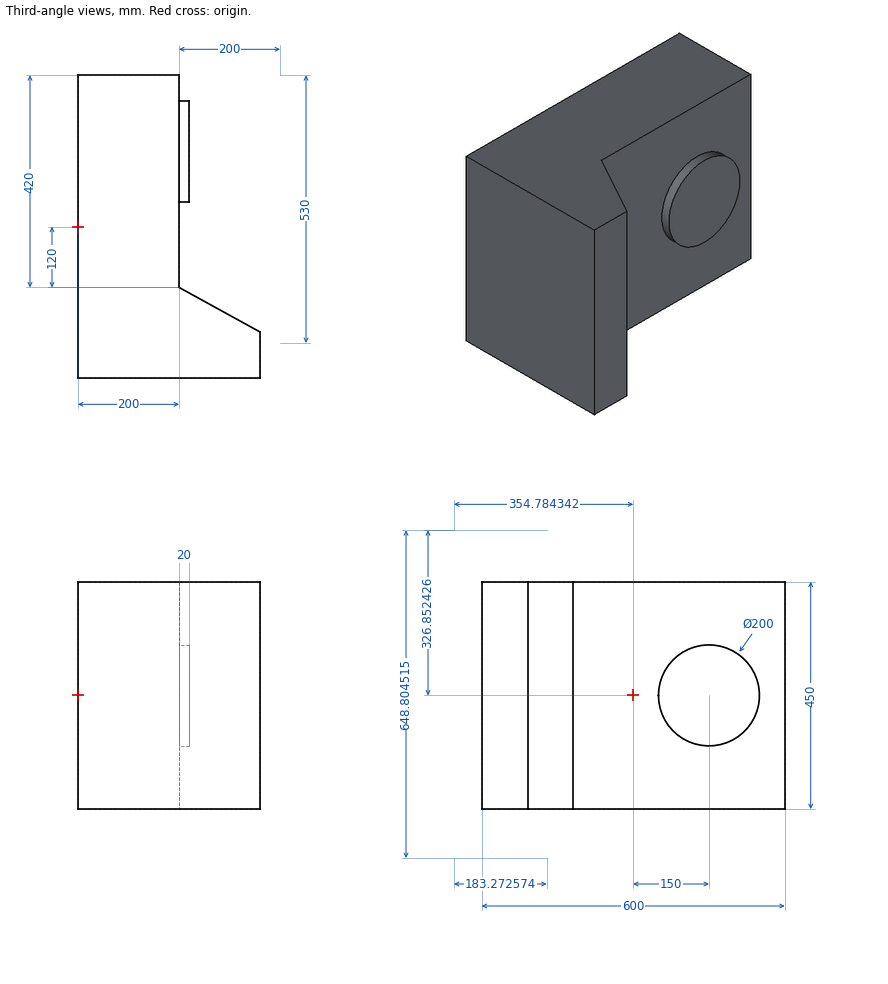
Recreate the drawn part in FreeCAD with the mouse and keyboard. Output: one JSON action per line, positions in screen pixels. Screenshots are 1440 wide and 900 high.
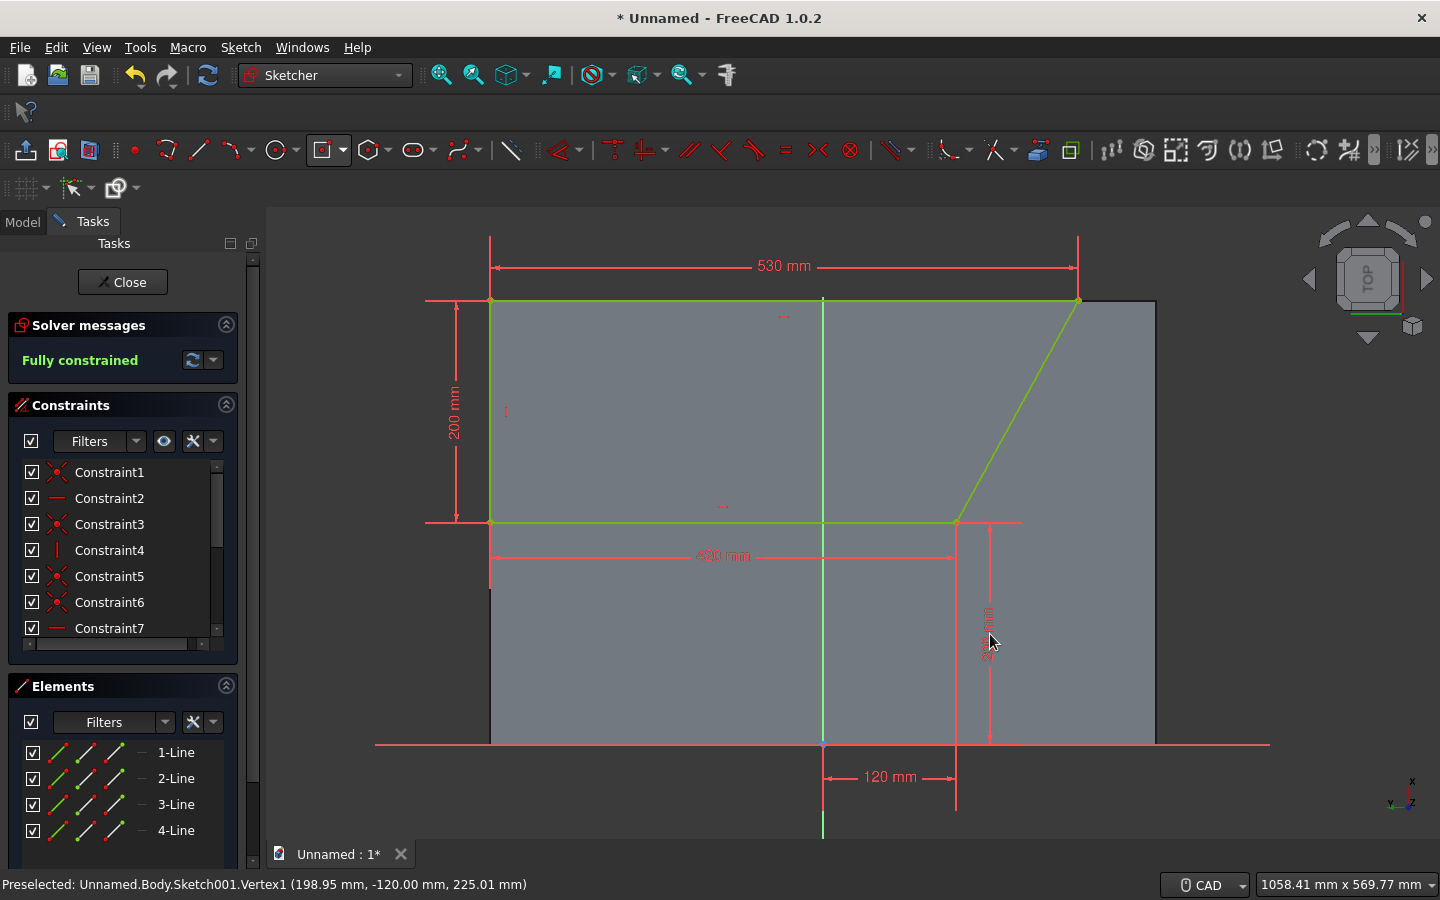
{"action": "left_click", "coordinate": [123, 282]}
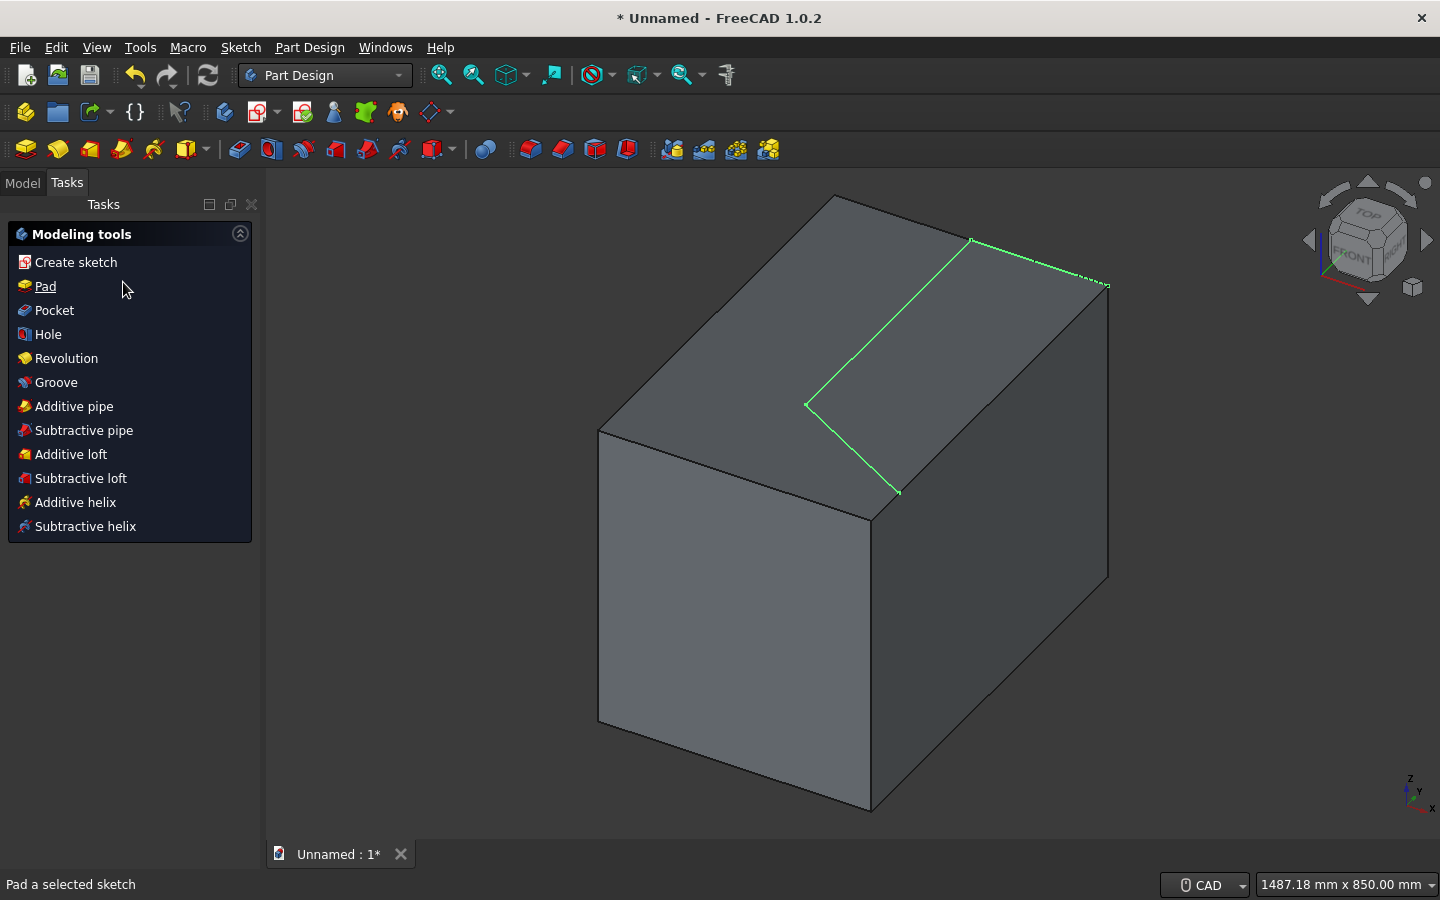
{"action": "left_click", "coordinate": [240, 150]}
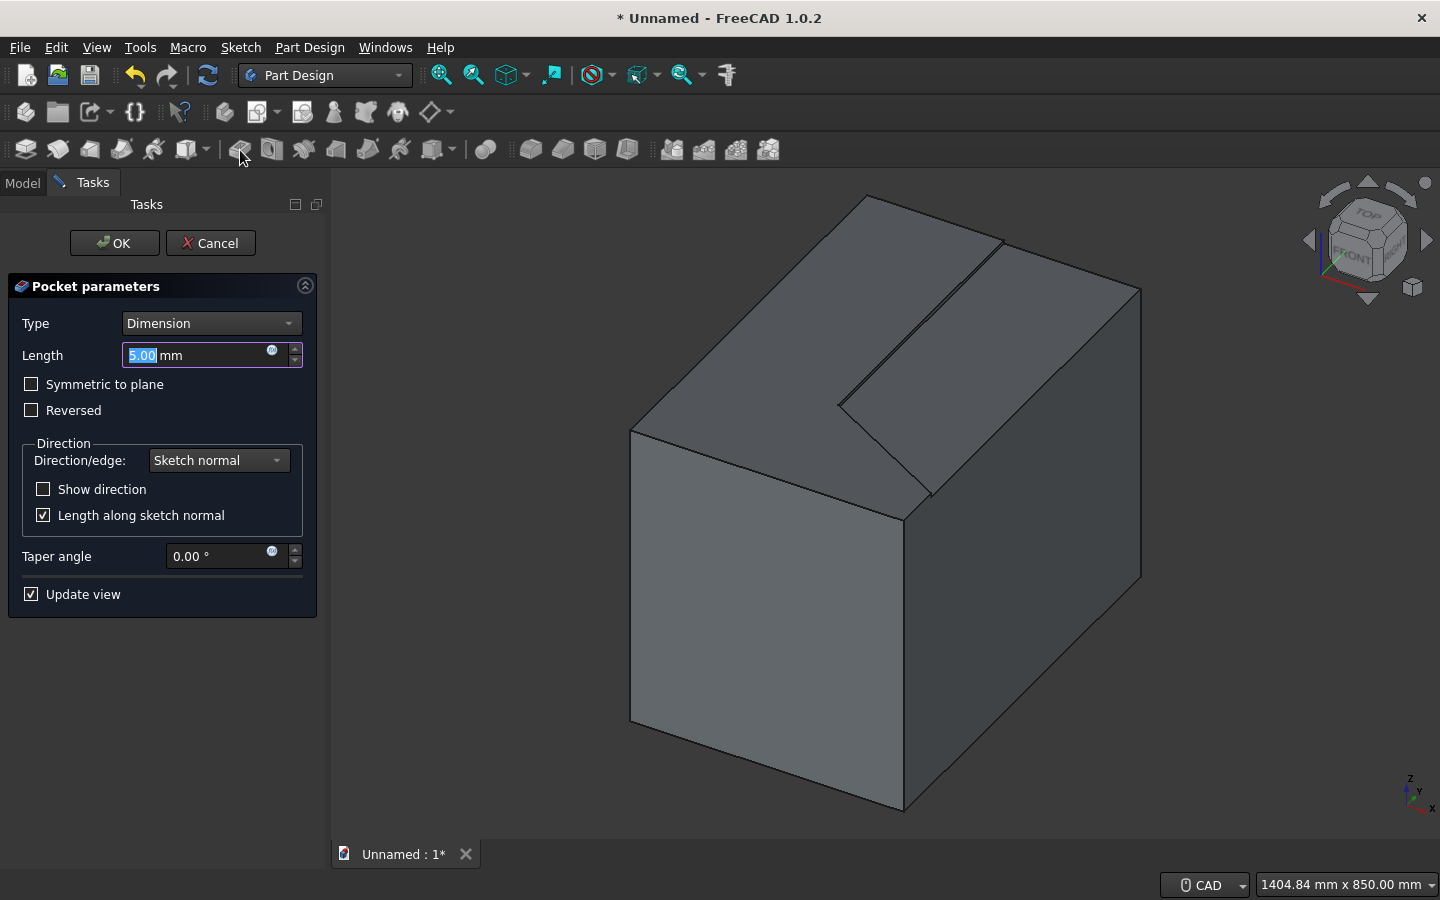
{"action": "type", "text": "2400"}
{"action": "key", "text": "Tab"}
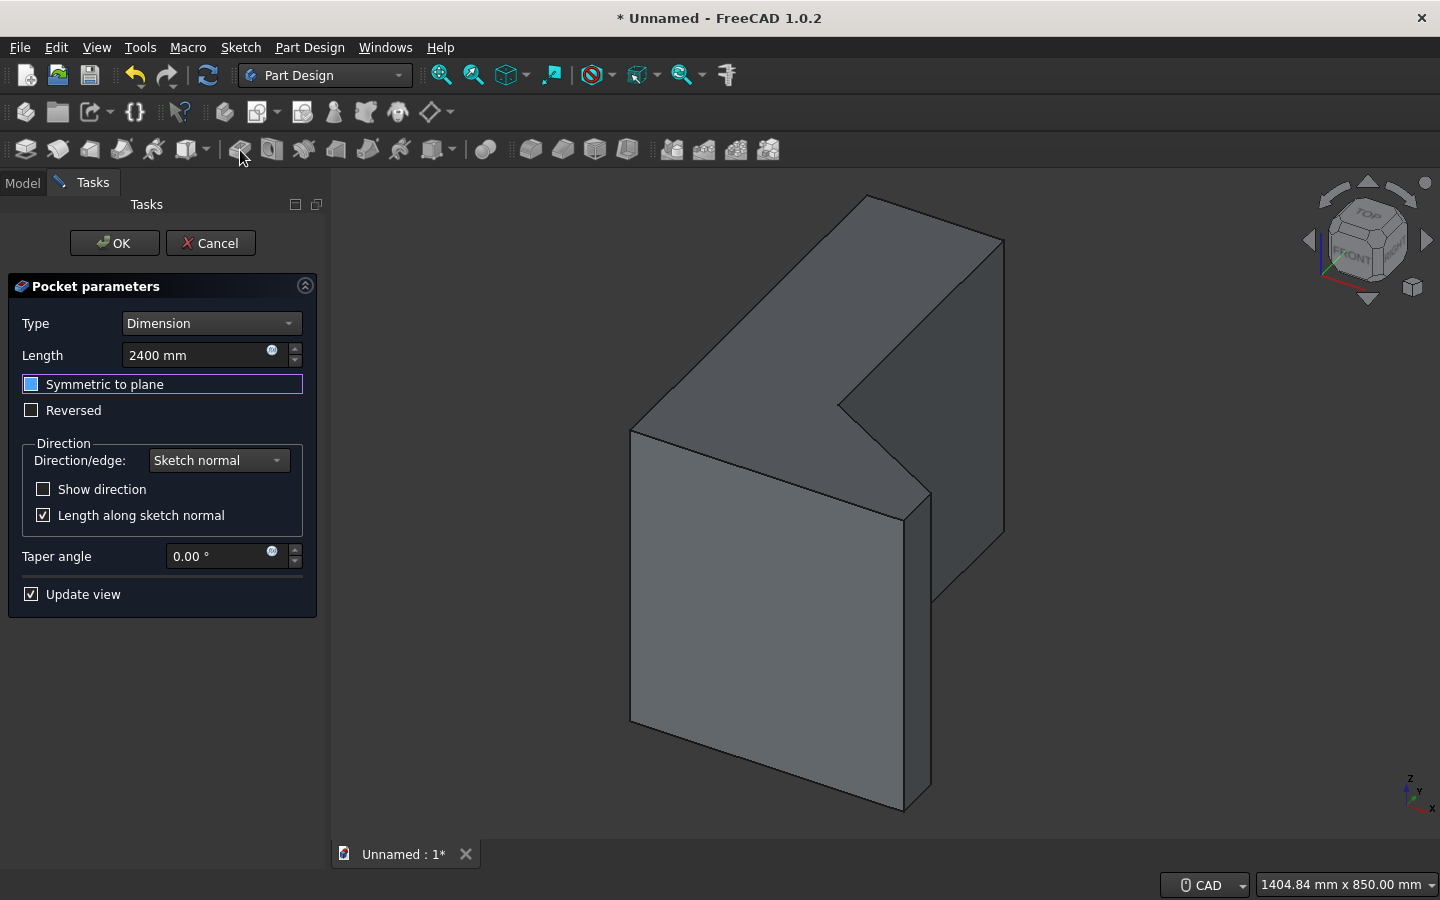
{"action": "left_click", "coordinate": [115, 243]}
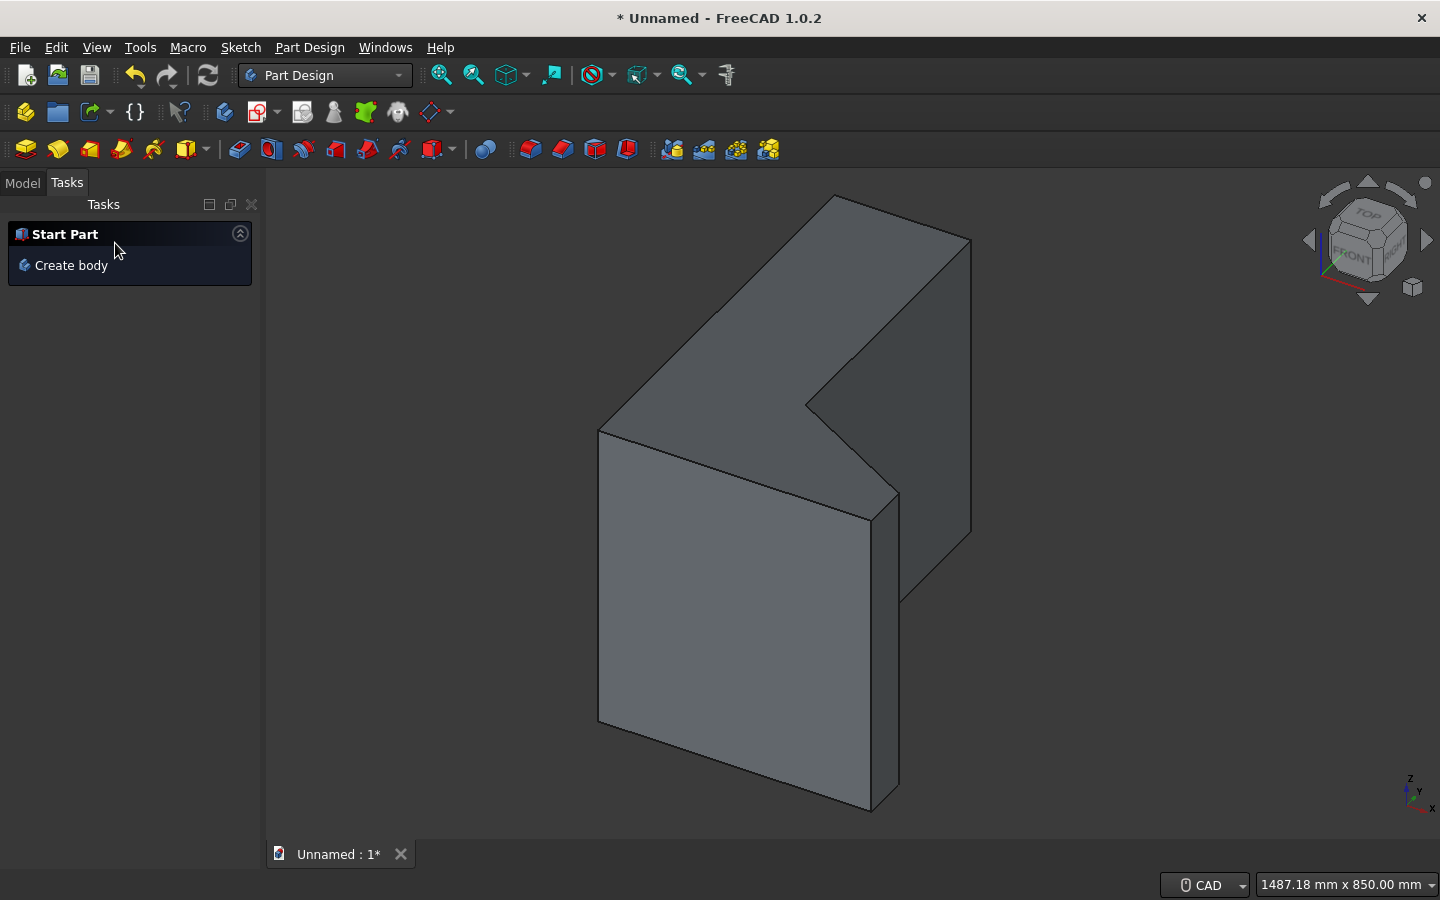
{"action": "left_click", "coordinate": [885, 693]}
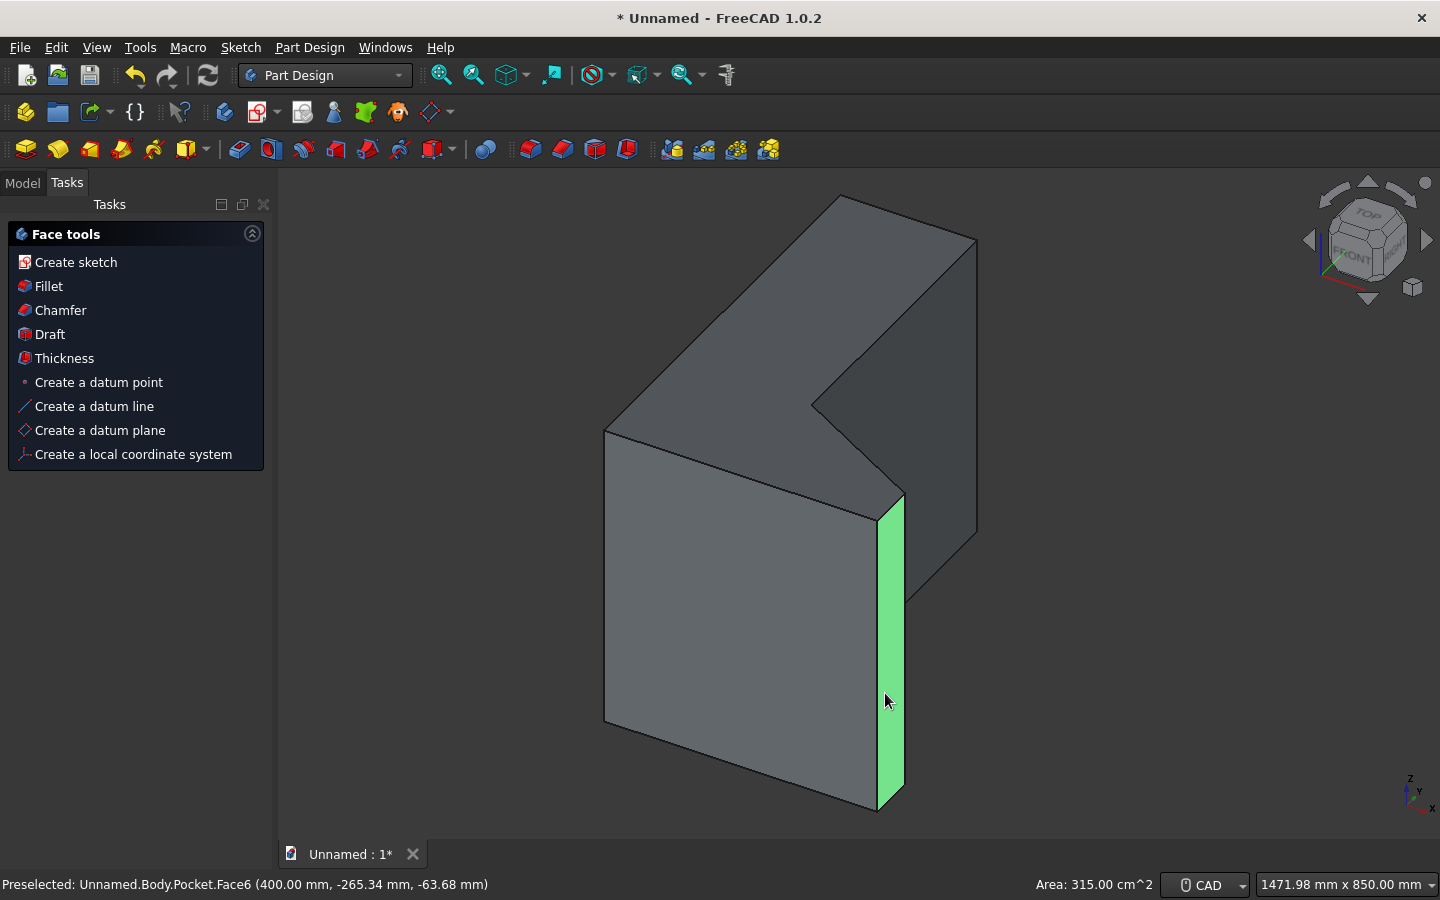
{"action": "left_click", "coordinate": [258, 112]}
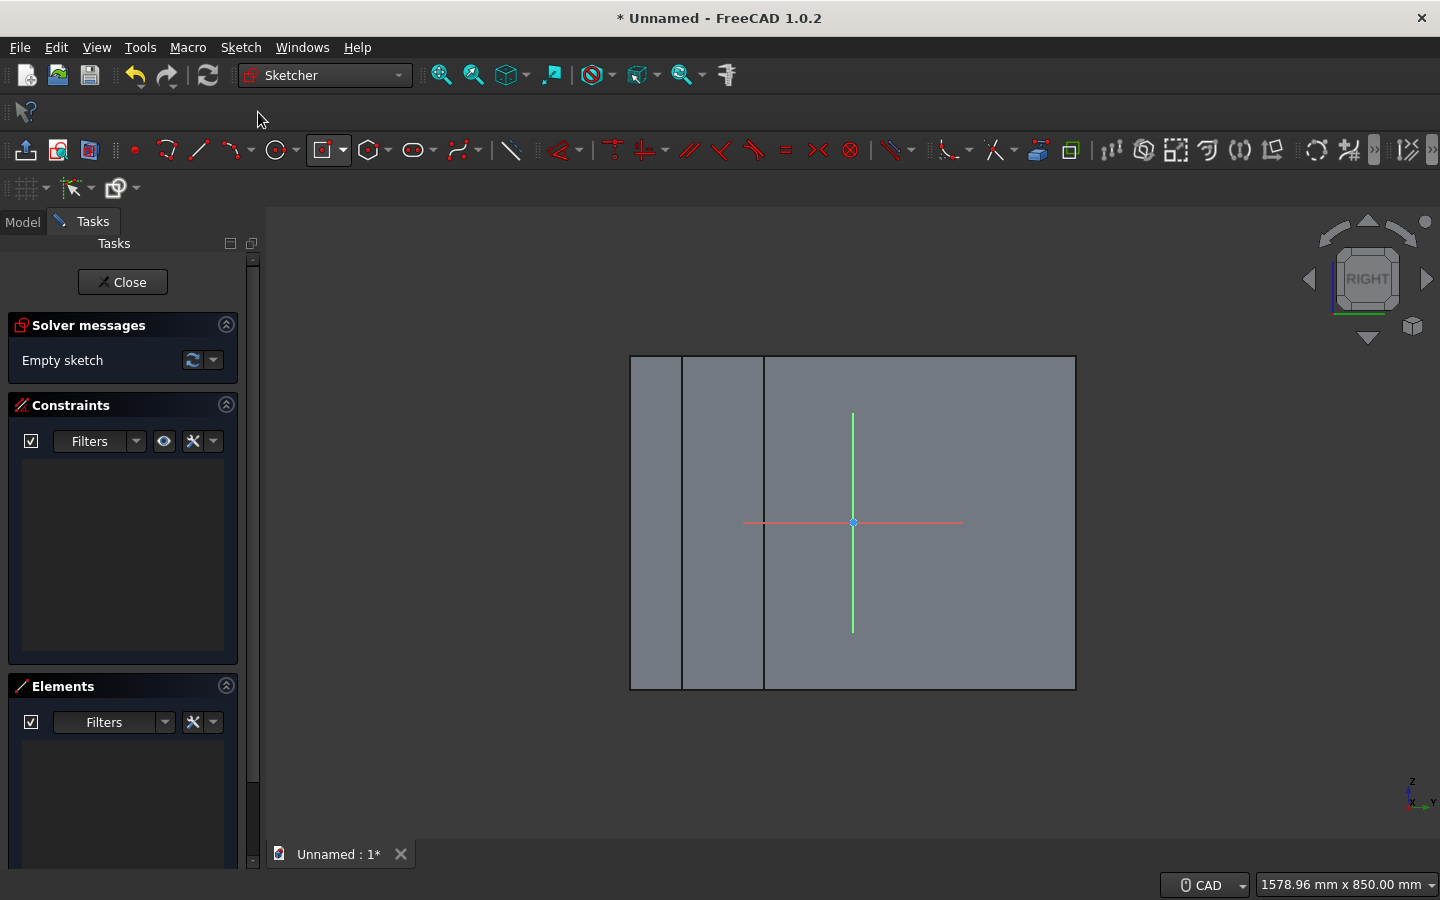
{"action": "key", "text": "g r"}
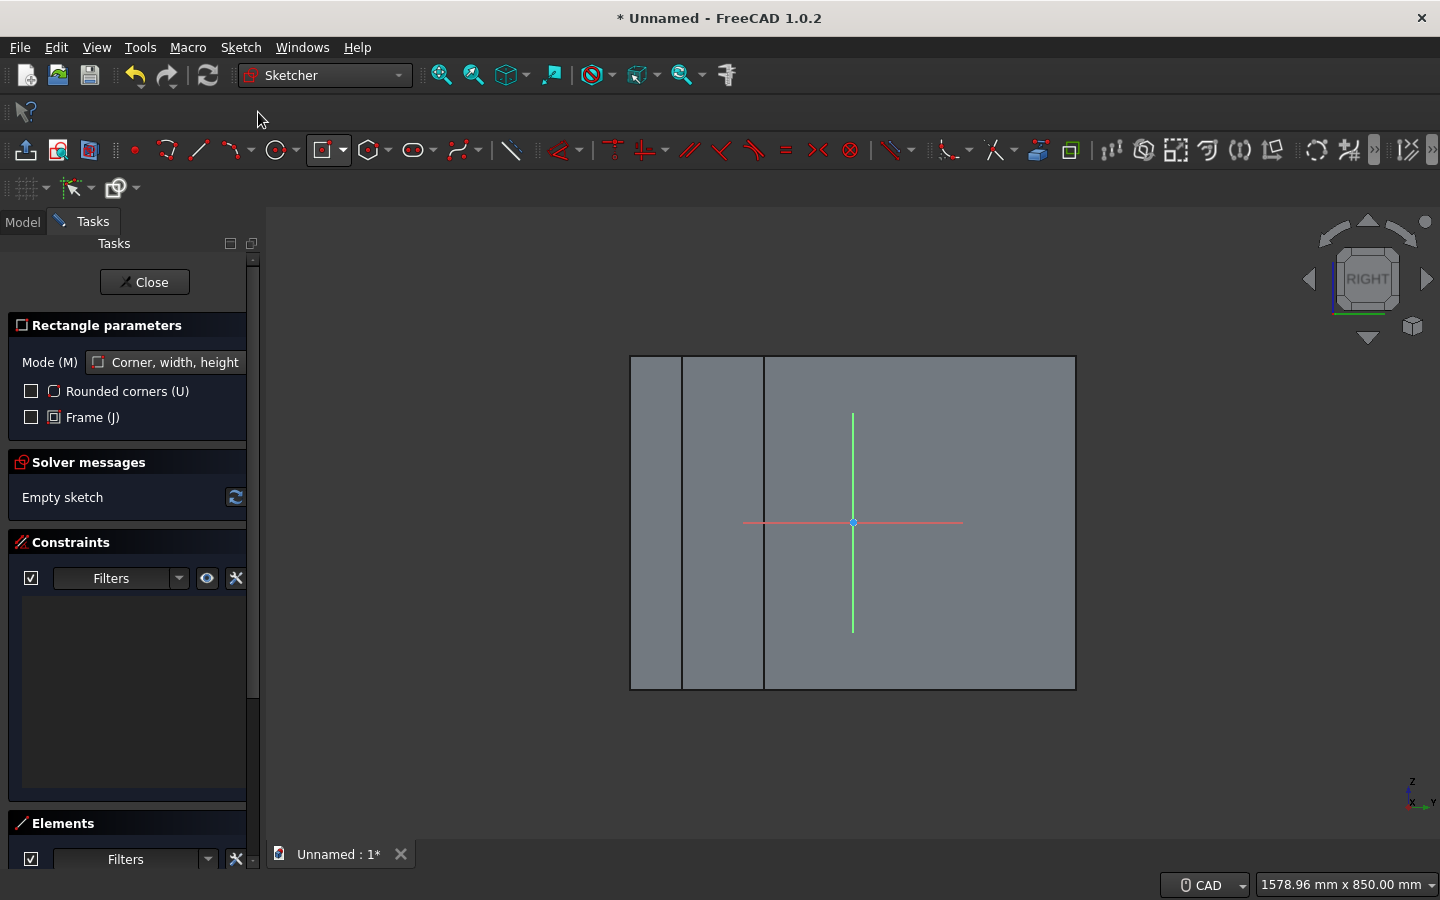
{"action": "left_click", "coordinate": [589, 280]}
{"action": "mouse_move", "coordinate": [725, 762]}